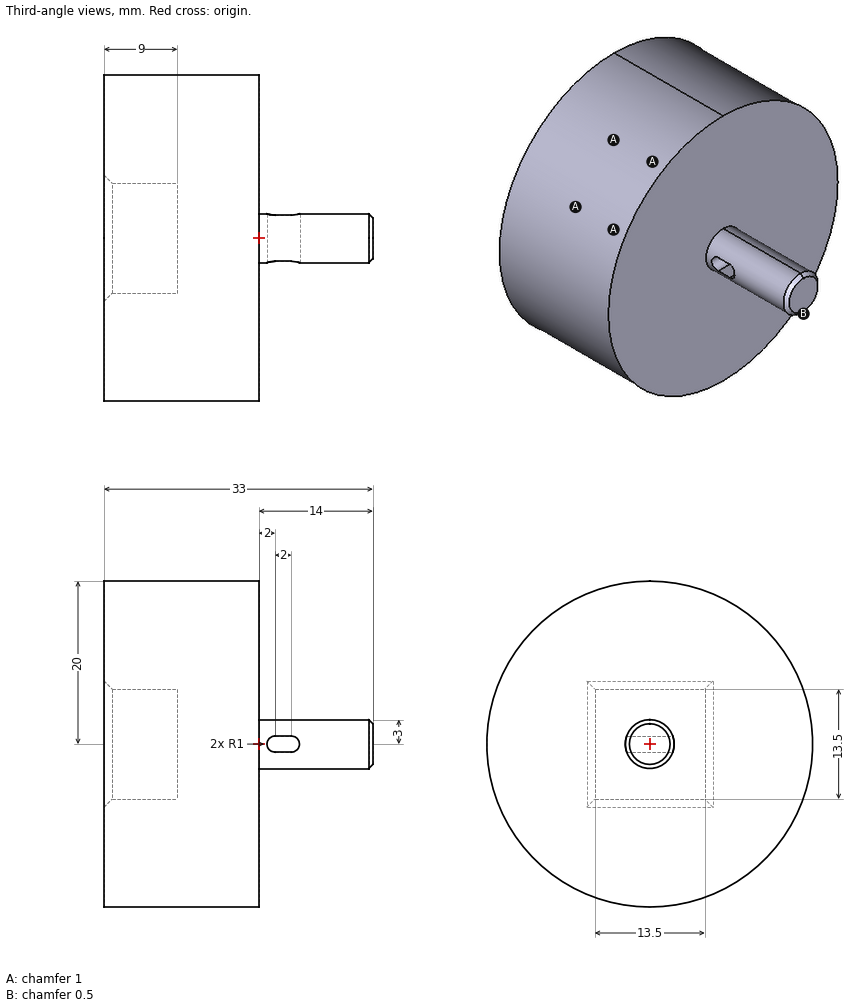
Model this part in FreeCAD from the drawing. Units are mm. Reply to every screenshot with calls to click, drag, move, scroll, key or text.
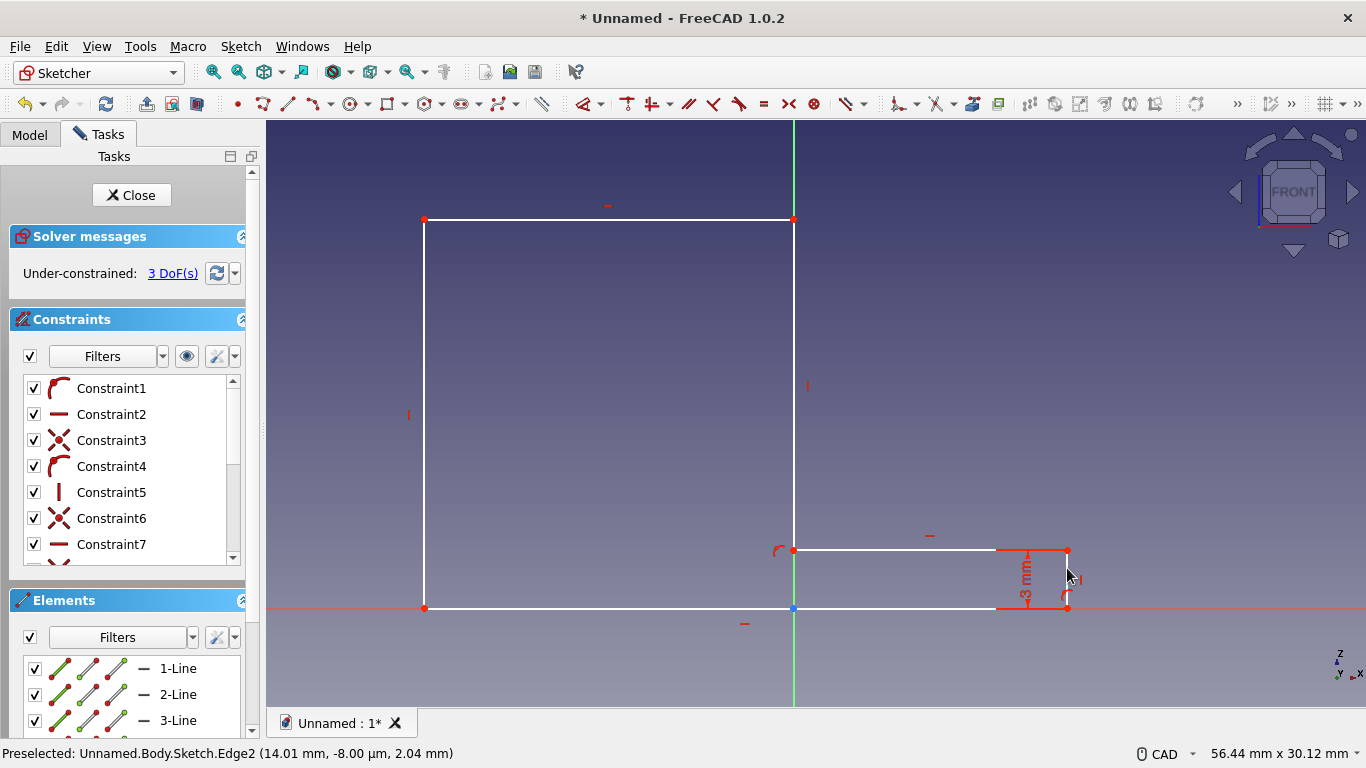
click(876, 550)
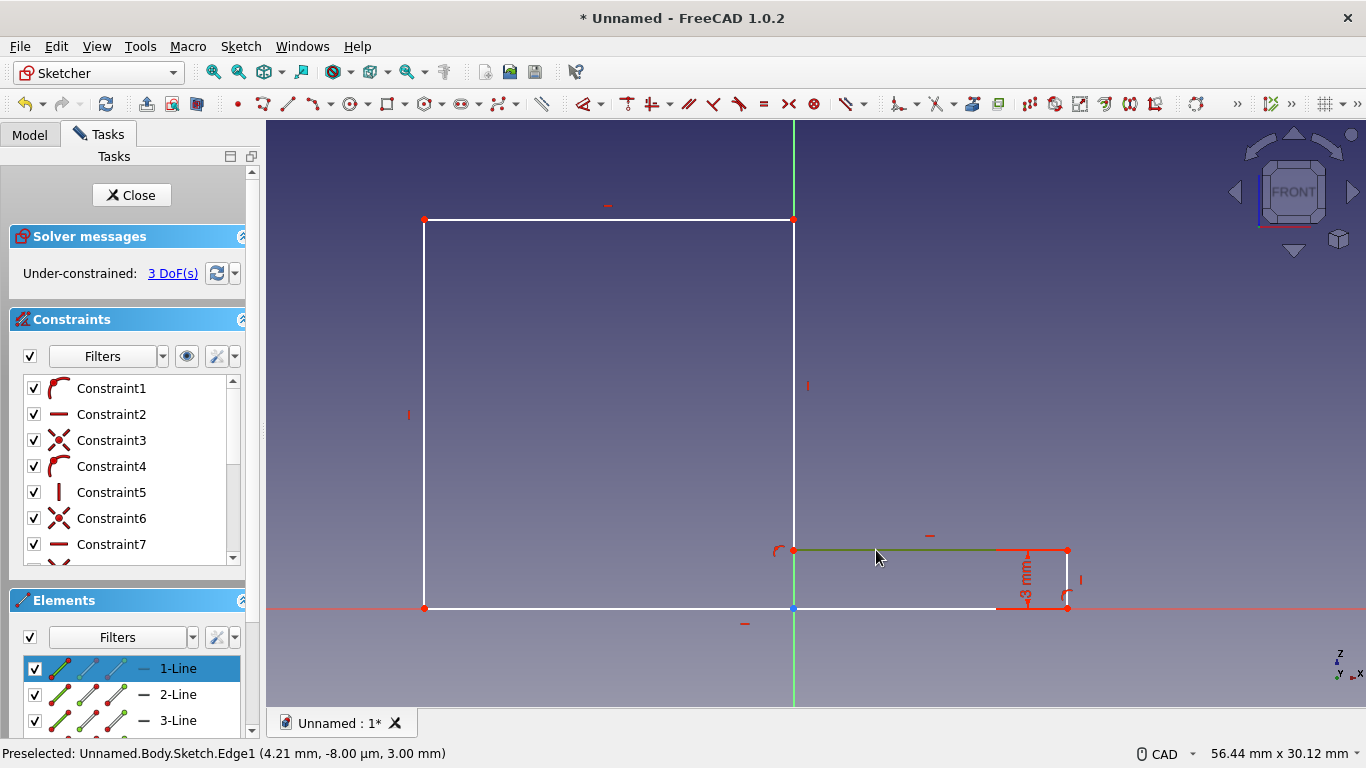
click(600, 104)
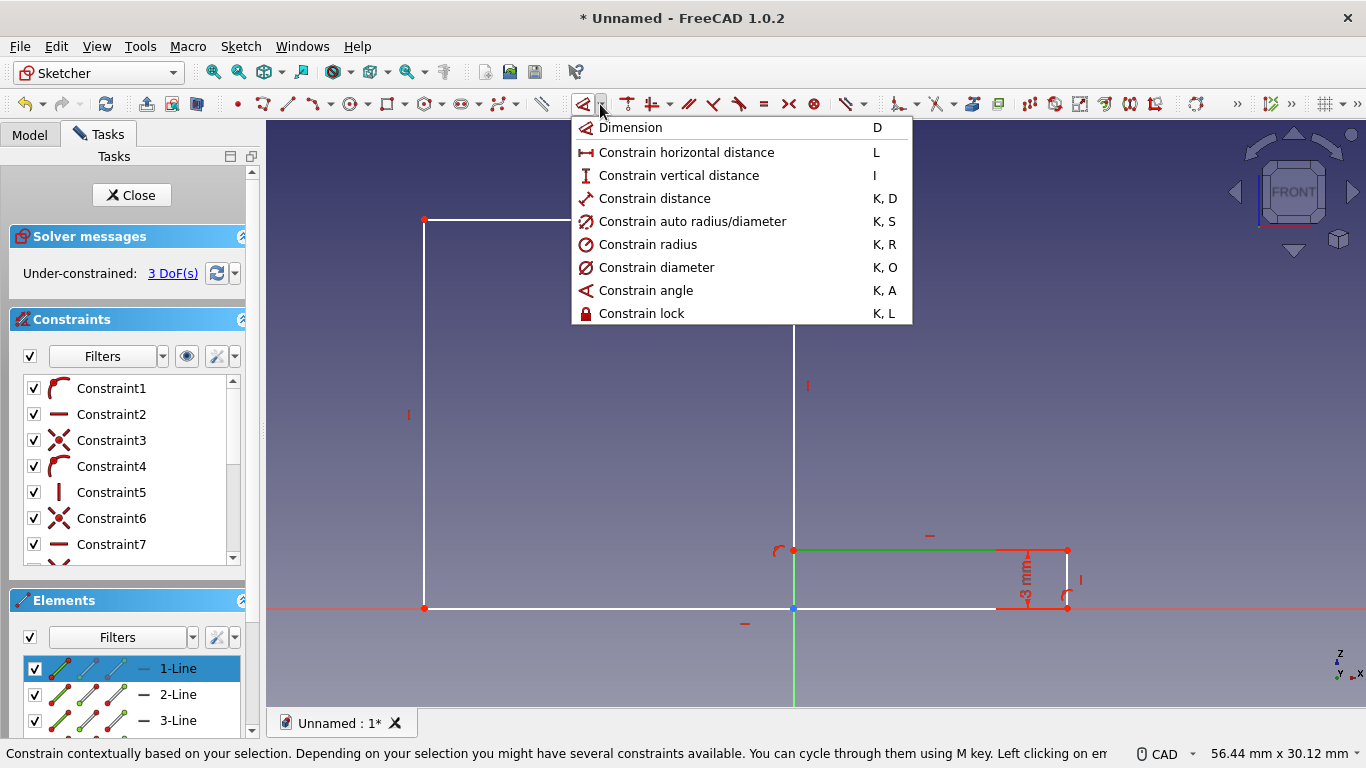
click(742, 152)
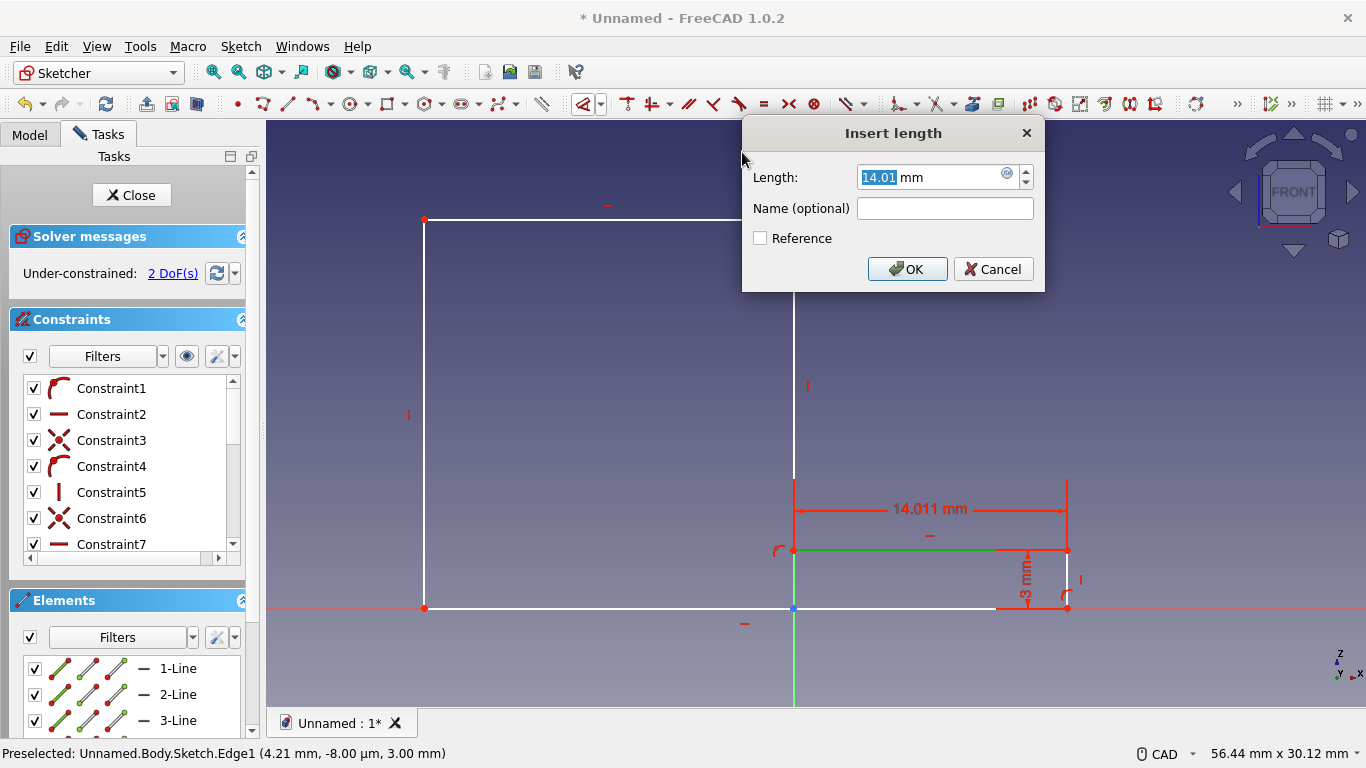
text(14)
key(Return)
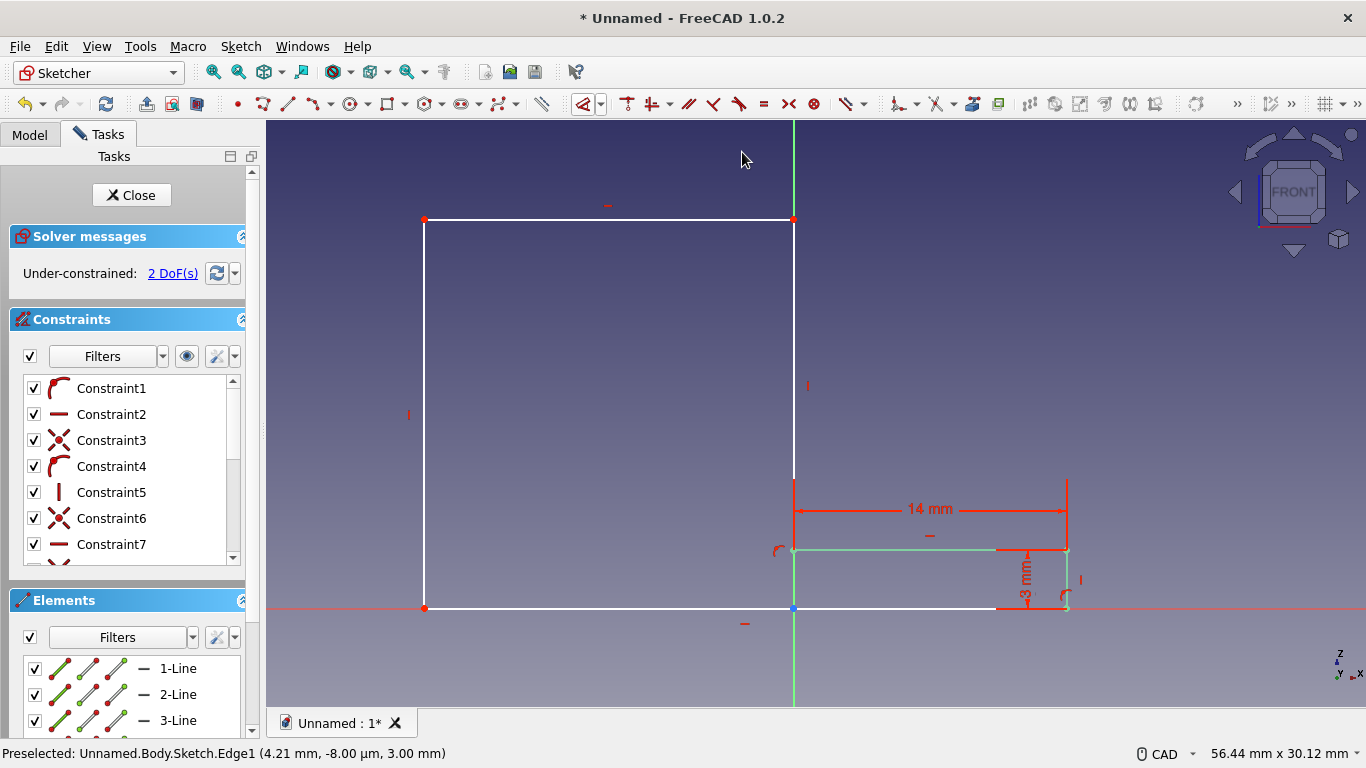
click(874, 609)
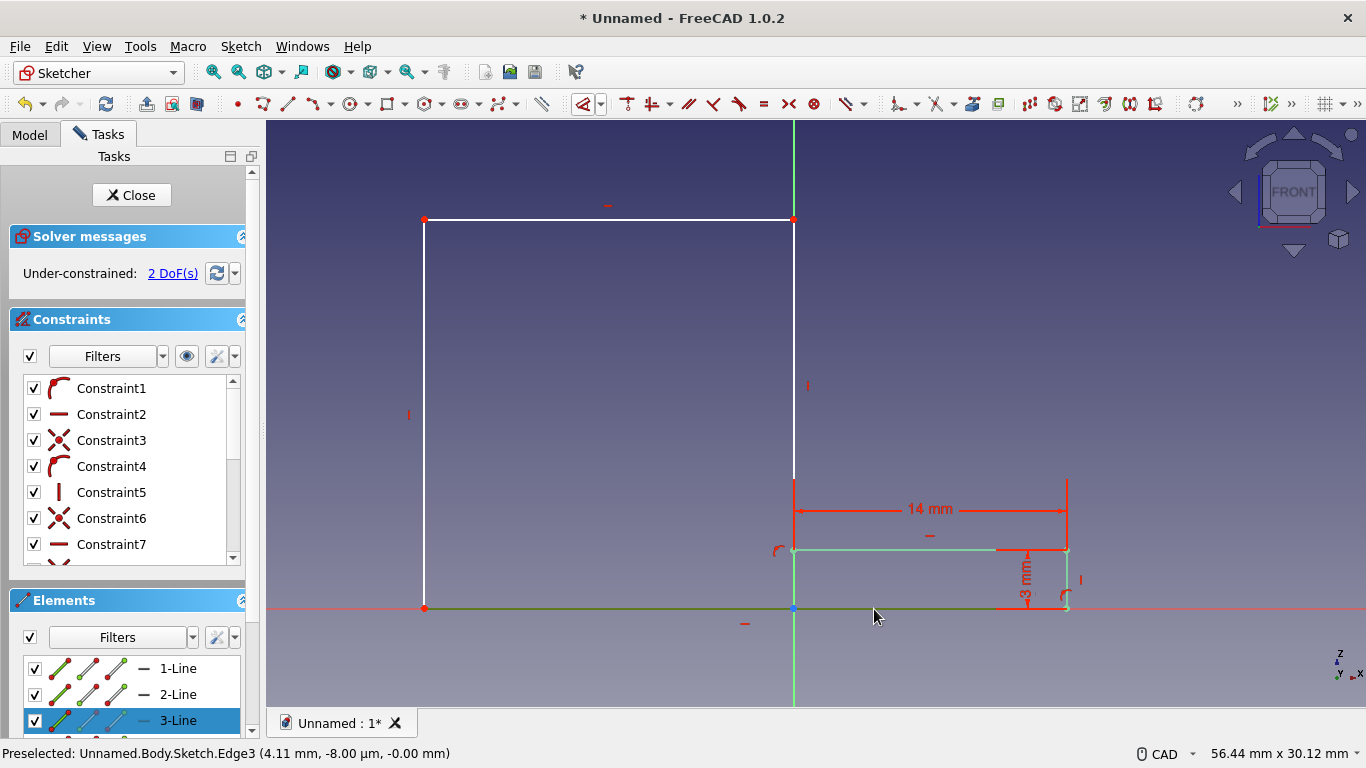
click(600, 104)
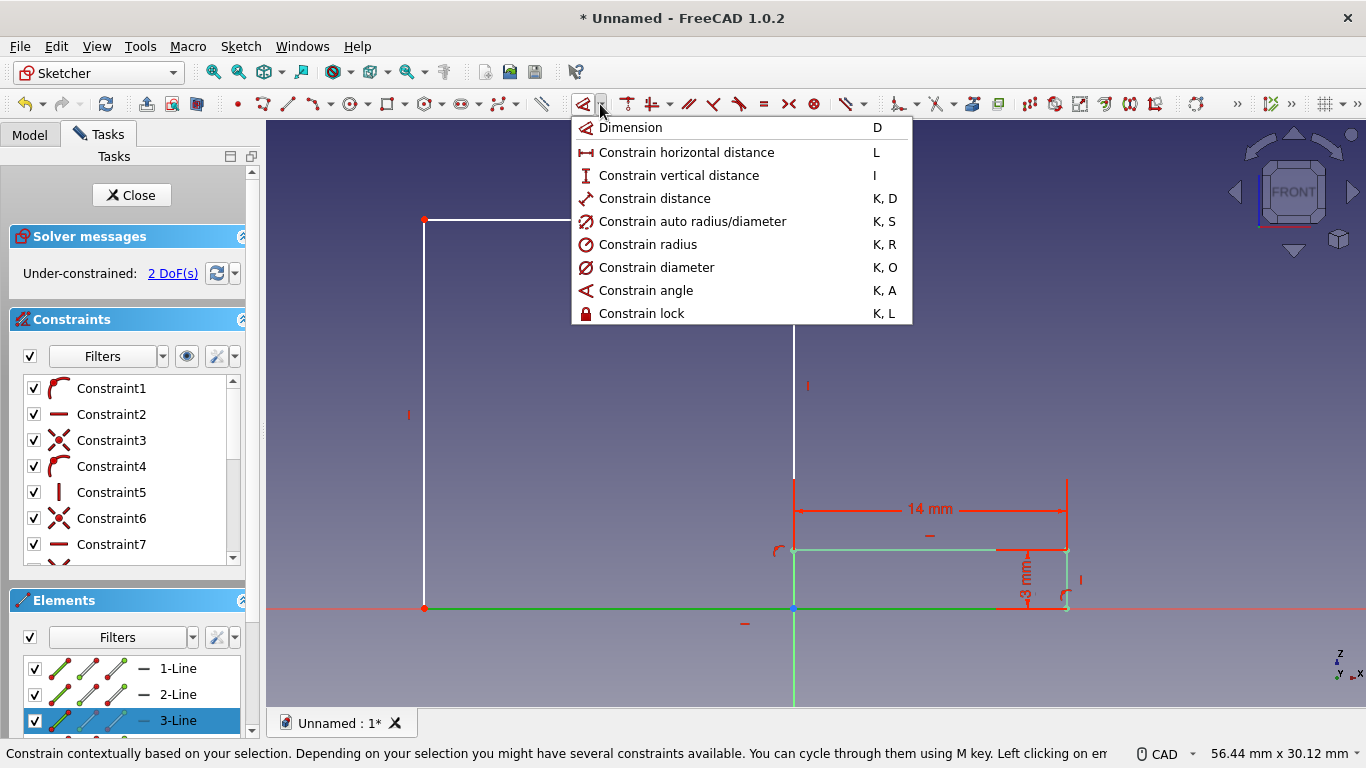
click(742, 152)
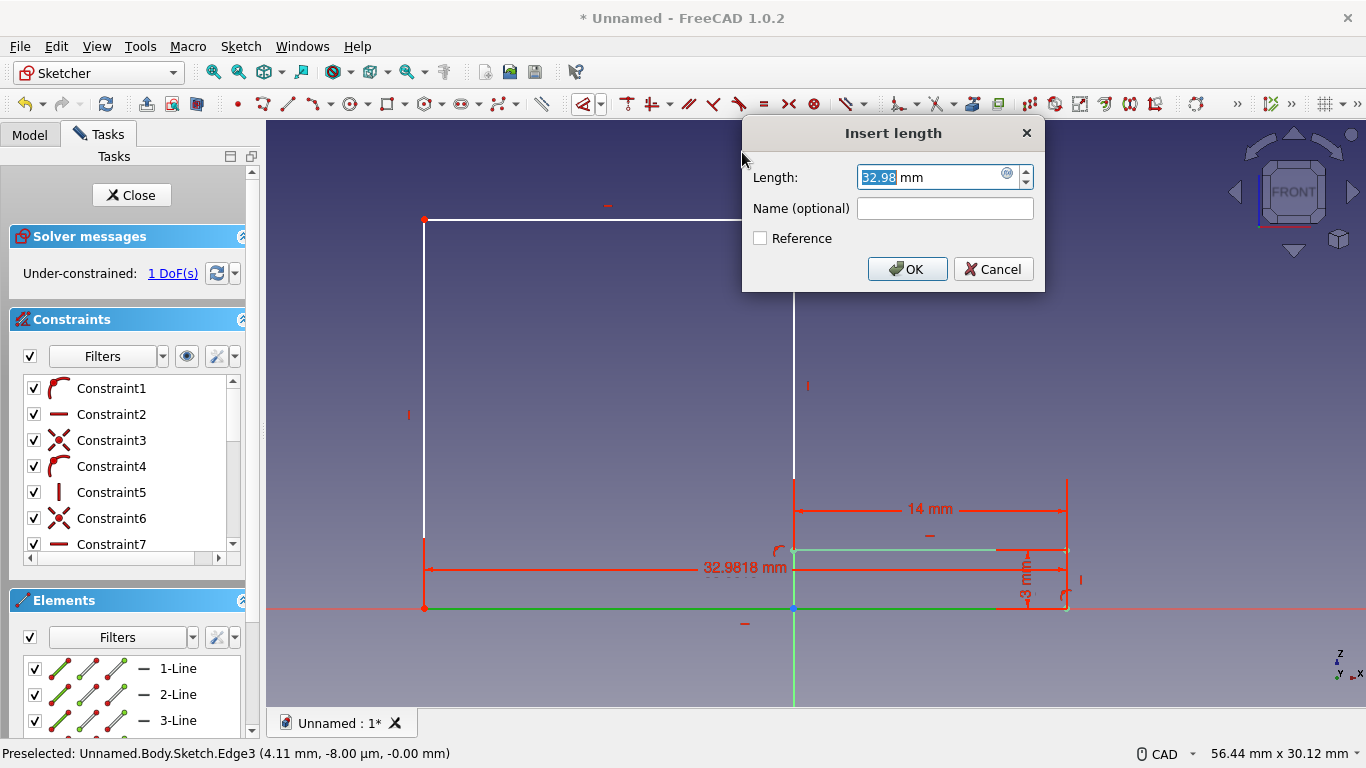
text(33)
key(Return)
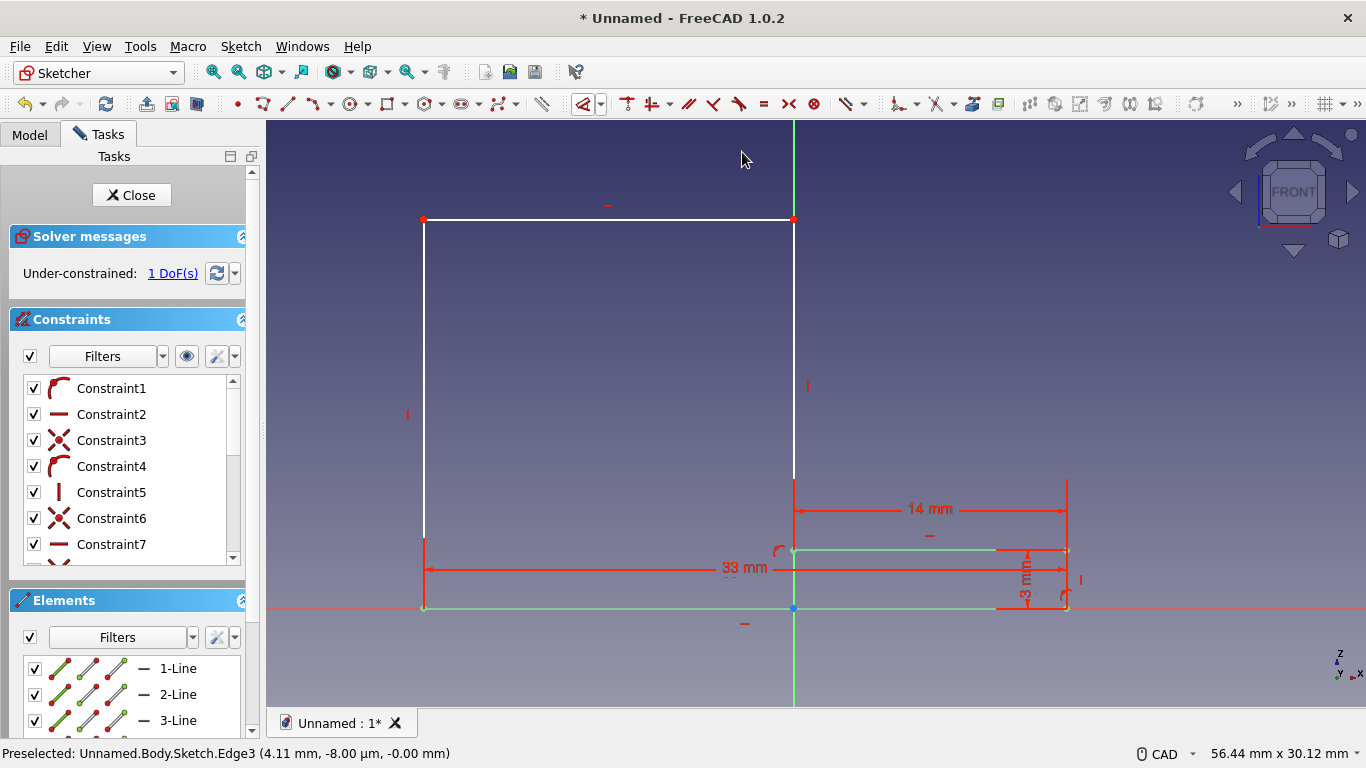
click(424, 492)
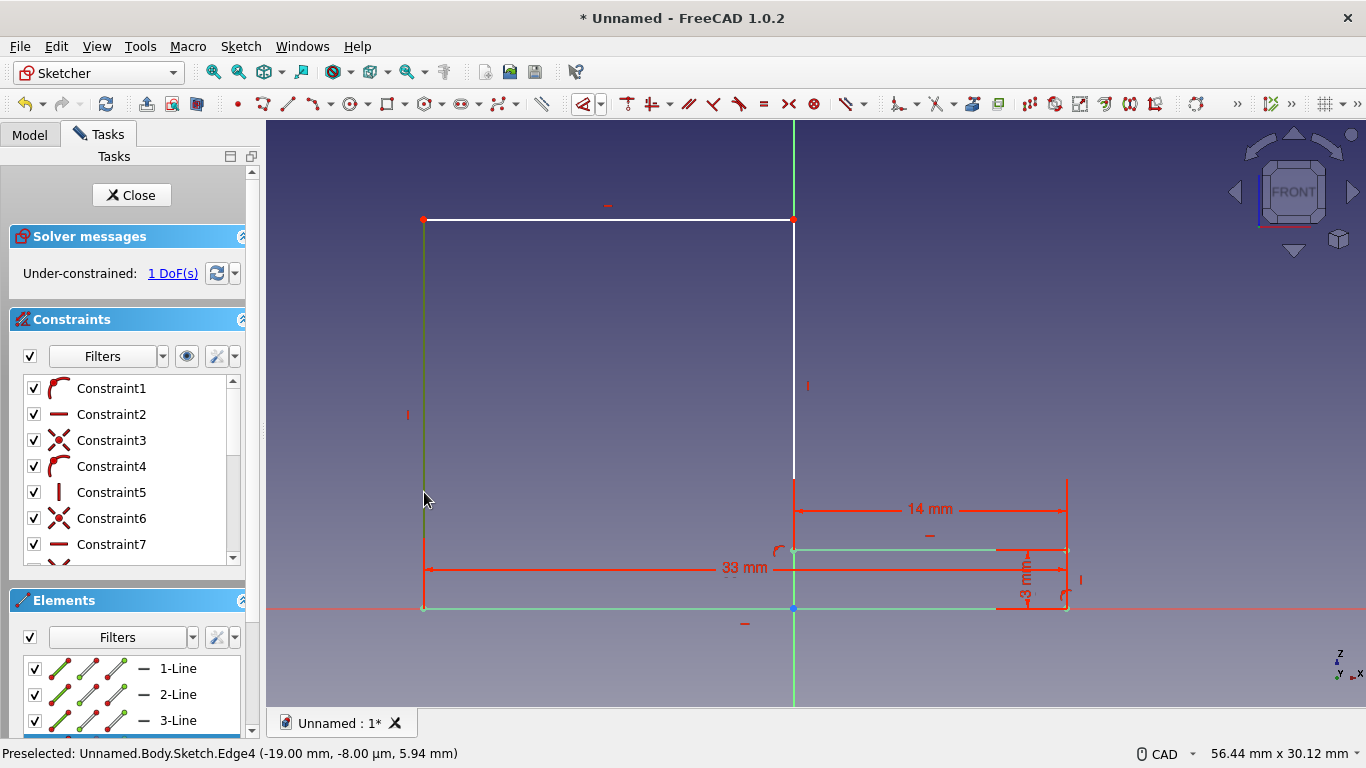
click(600, 104)